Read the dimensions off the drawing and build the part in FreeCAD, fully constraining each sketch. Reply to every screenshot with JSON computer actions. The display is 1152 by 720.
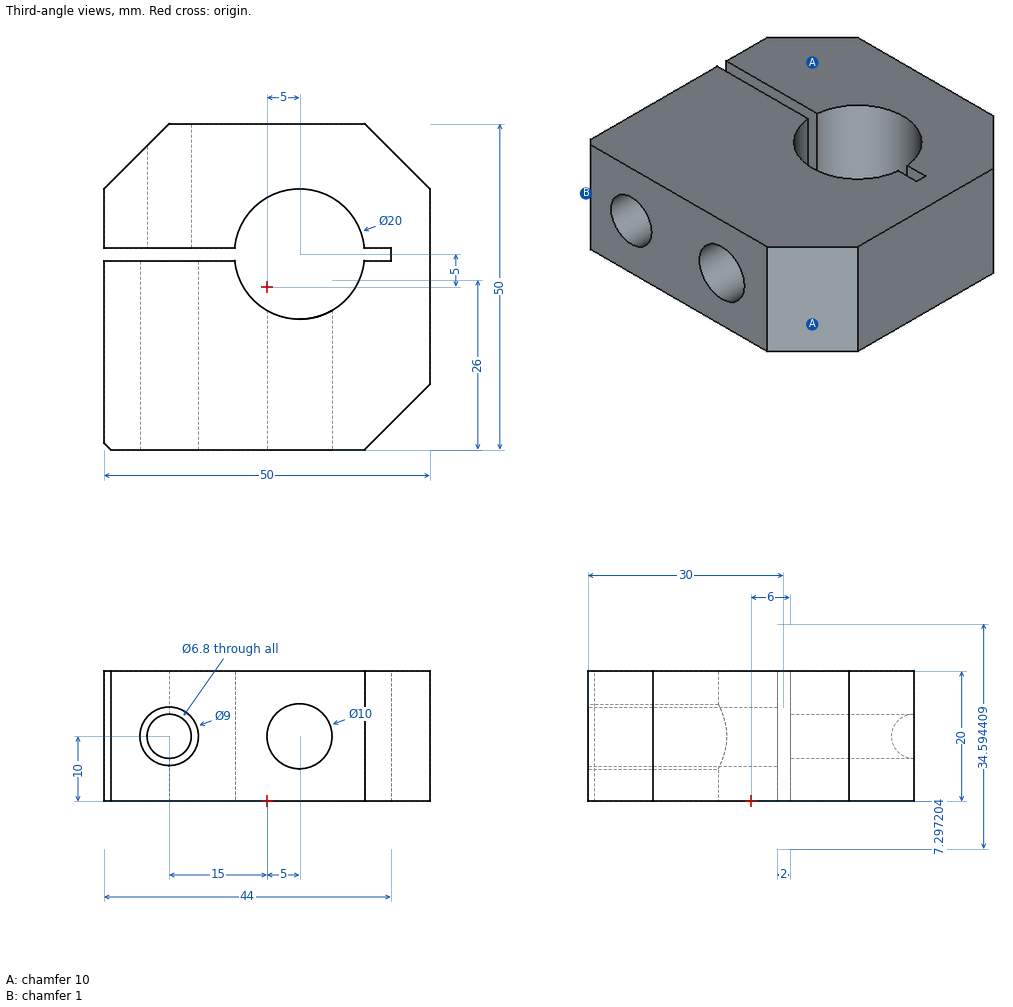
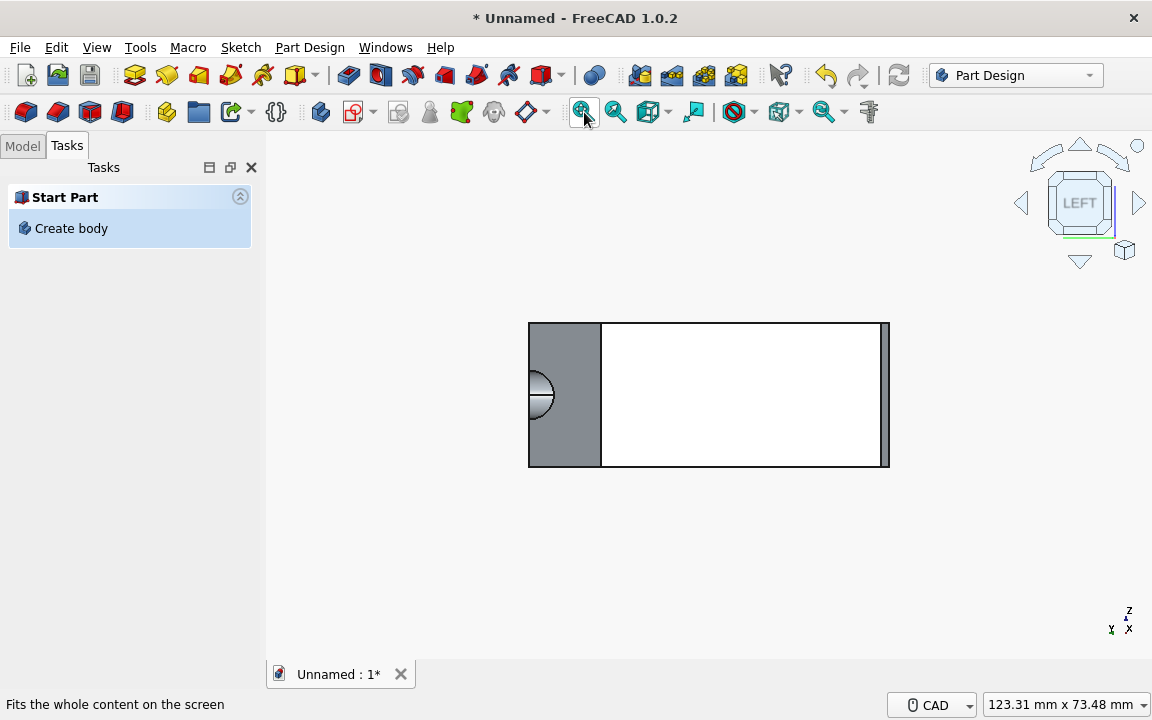
{"action": "left_click", "coordinate": [701, 394]}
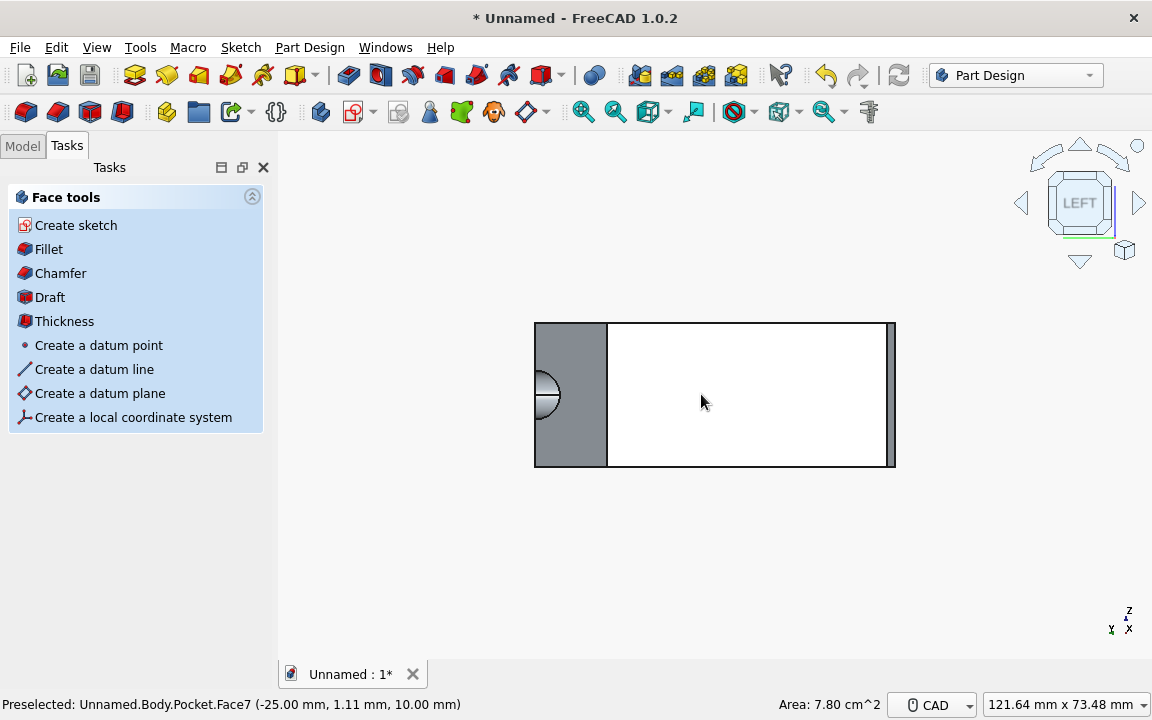
{"action": "left_click", "coordinate": [354, 112]}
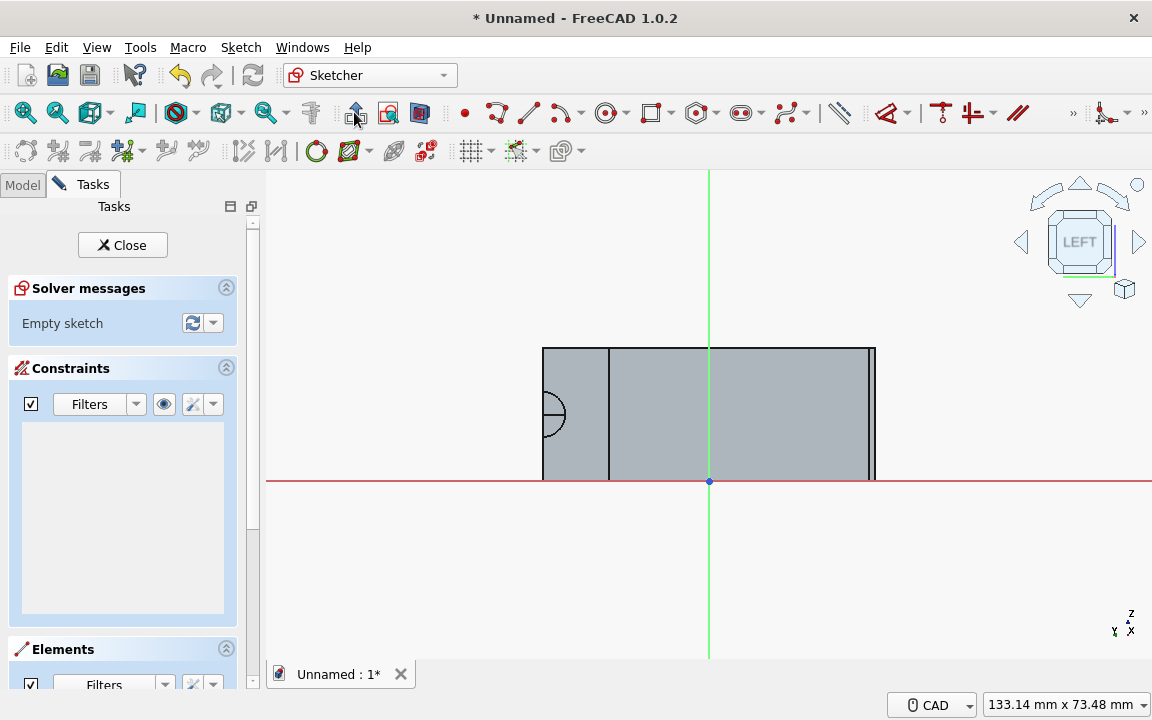
{"action": "left_click", "coordinate": [652, 114]}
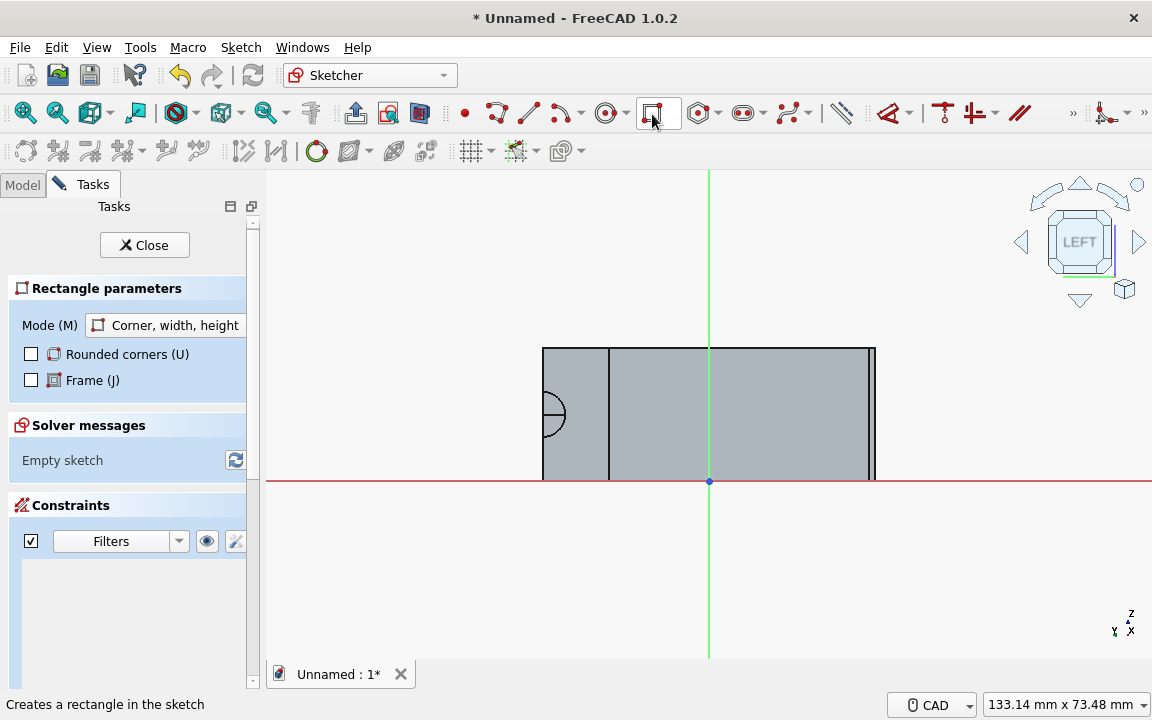
{"action": "left_click", "coordinate": [669, 299]}
{"action": "mouse_move", "coordinate": [682, 530]}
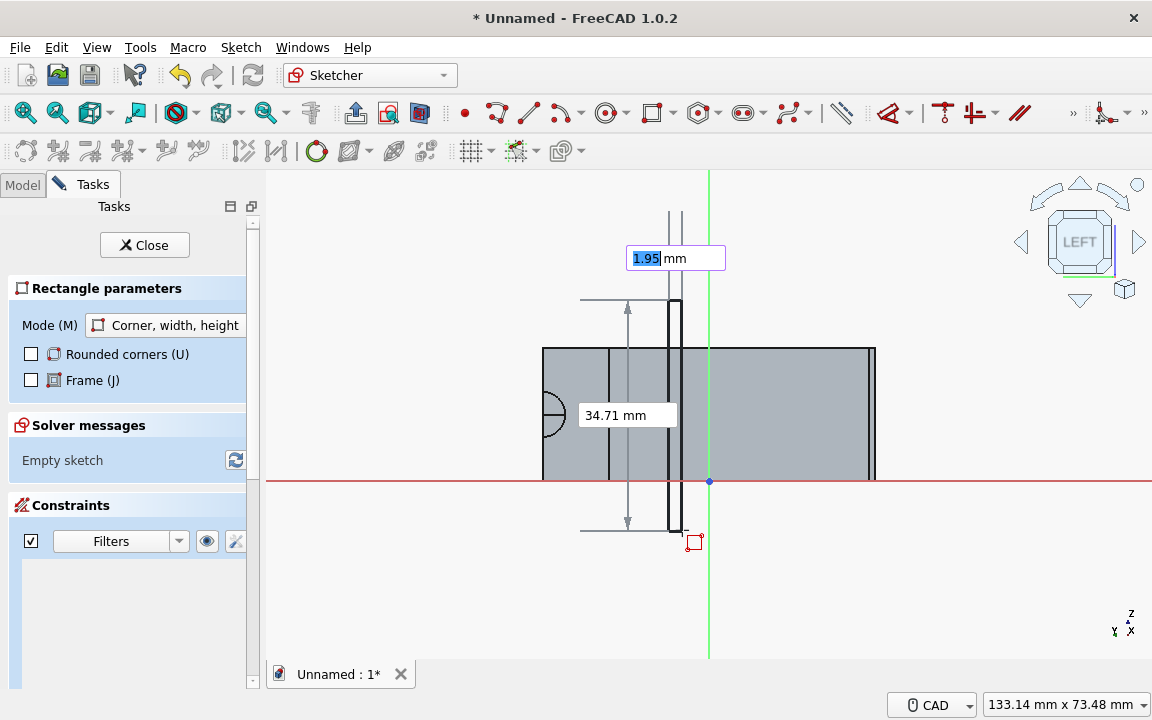
{"action": "type", "text": "2"}
{"action": "key", "text": "Tab"}
{"action": "type", "text": "34.594409"}
{"action": "key", "text": "Return"}
{"action": "key", "text": "Escape"}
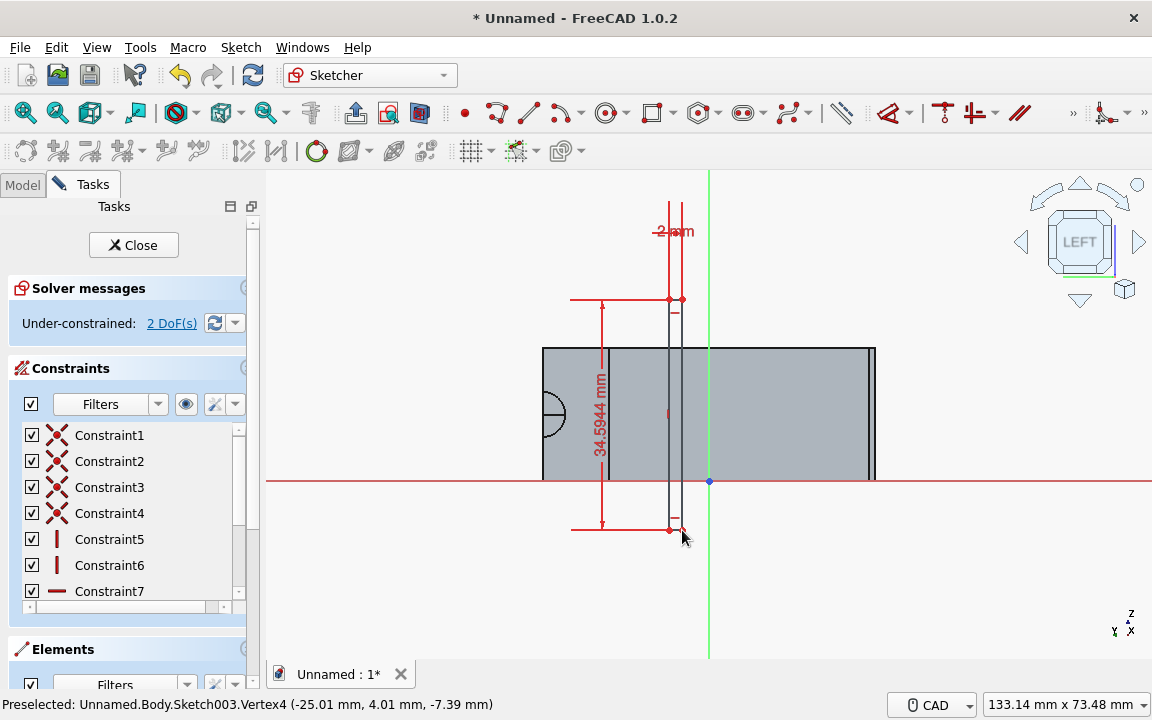
{"action": "left_click", "coordinate": [888, 114]}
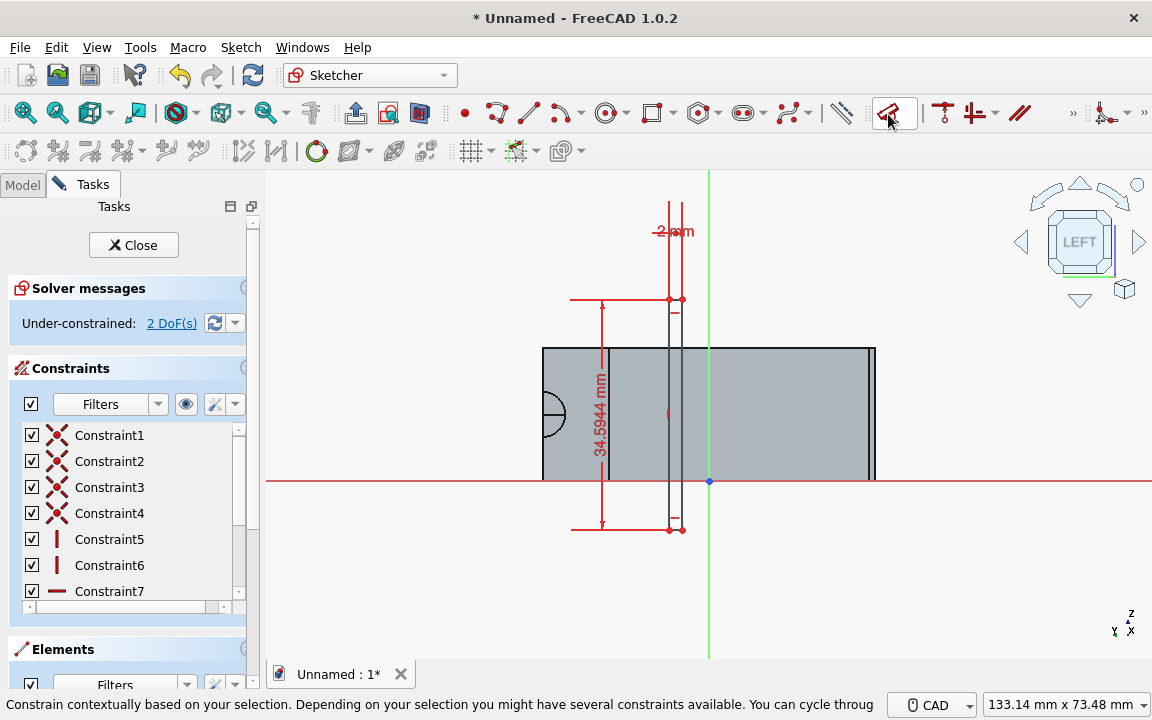
{"action": "left_click", "coordinate": [669, 300]}
{"action": "left_click", "coordinate": [689, 266]}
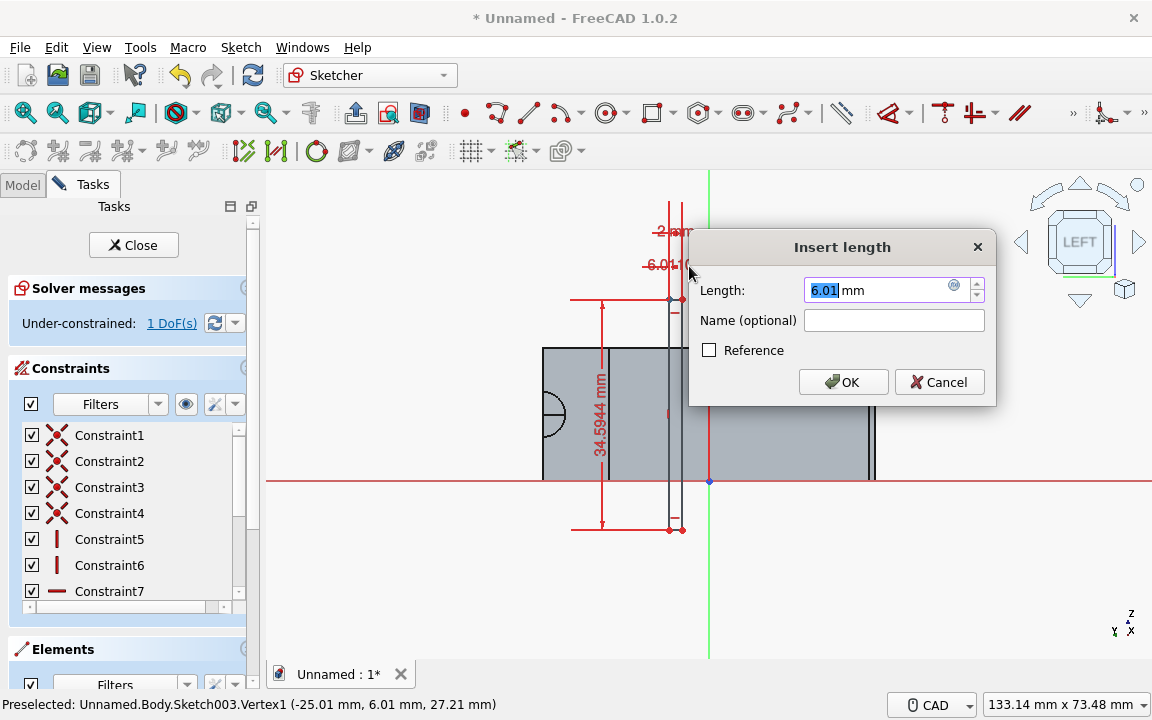
{"action": "type", "text": "6"}
{"action": "key", "text": "Return"}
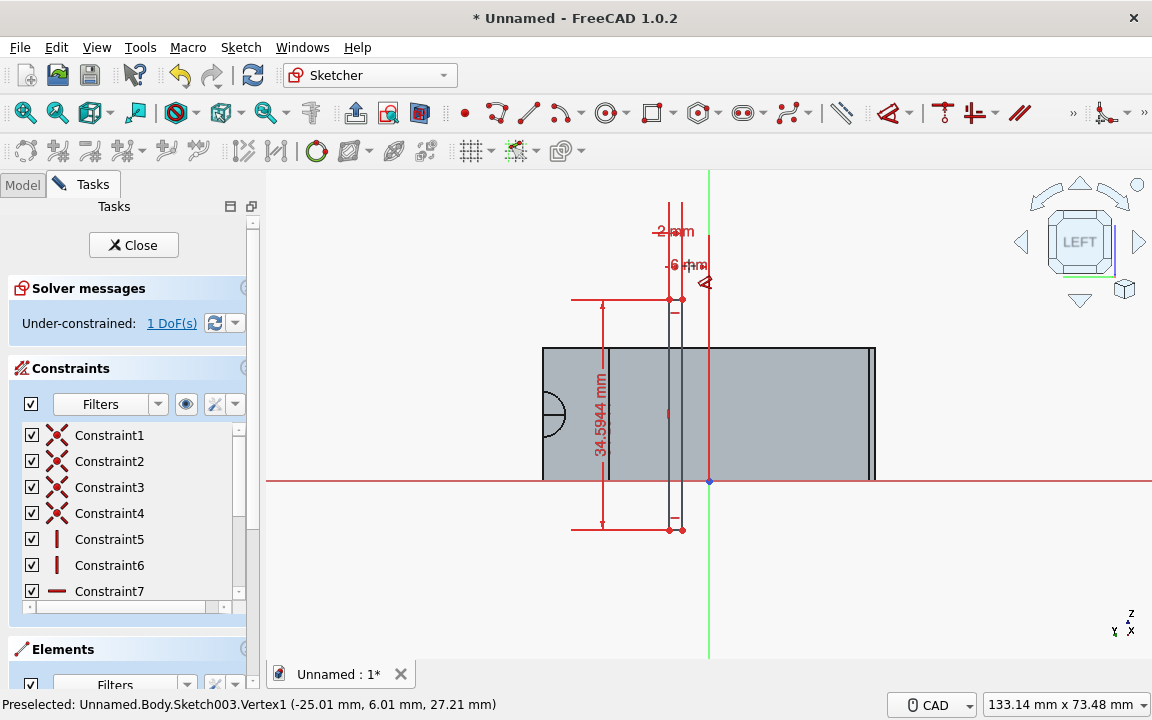
{"action": "left_click", "coordinate": [669, 530]}
{"action": "left_click", "coordinate": [743, 506]}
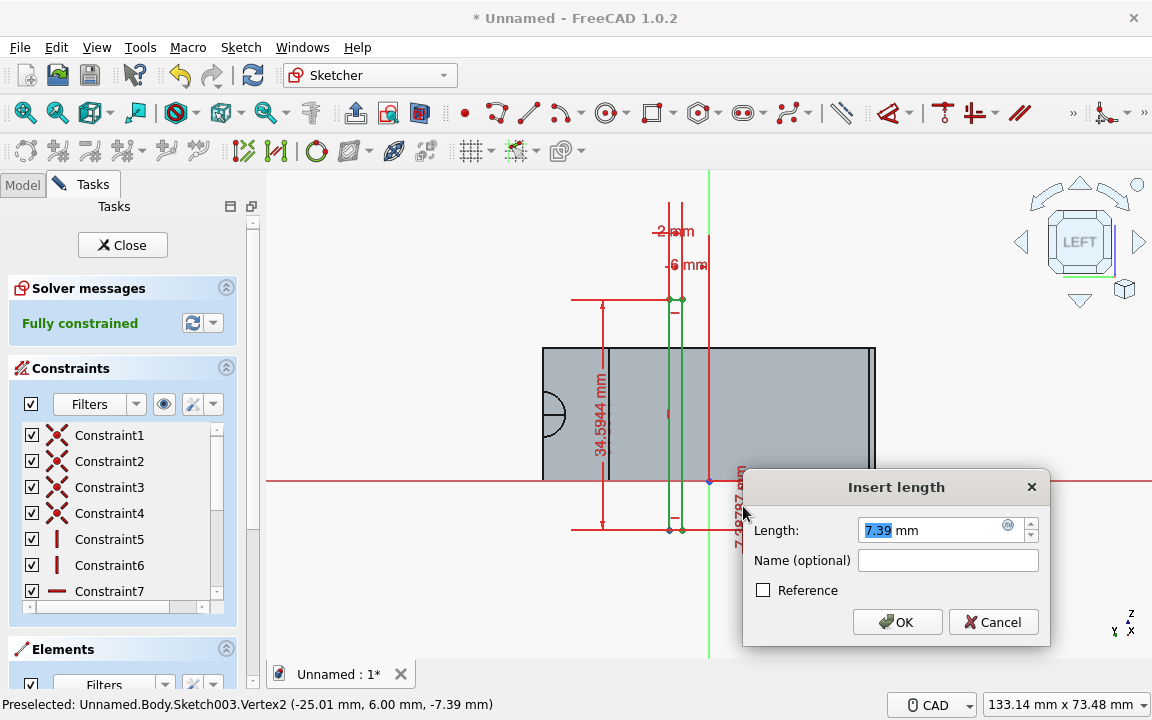
{"action": "type", "text": "7.297204"}
{"action": "key", "text": "Return"}
{"action": "key", "text": "Escape"}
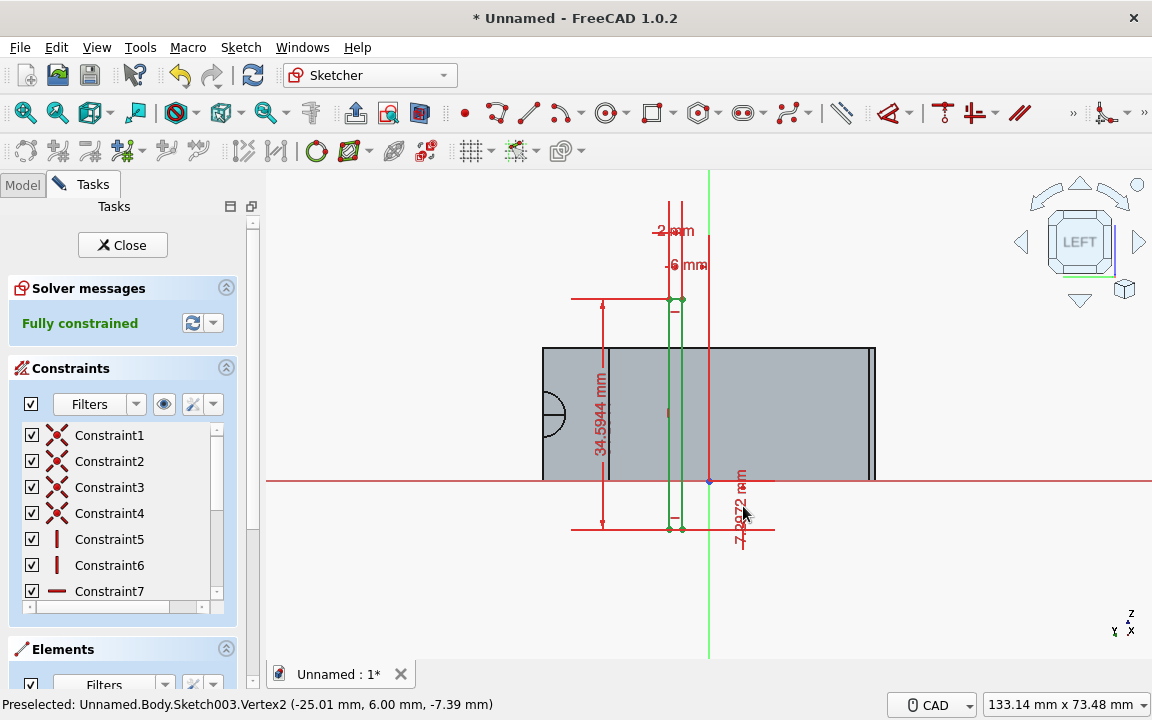
{"action": "left_click", "coordinate": [123, 245]}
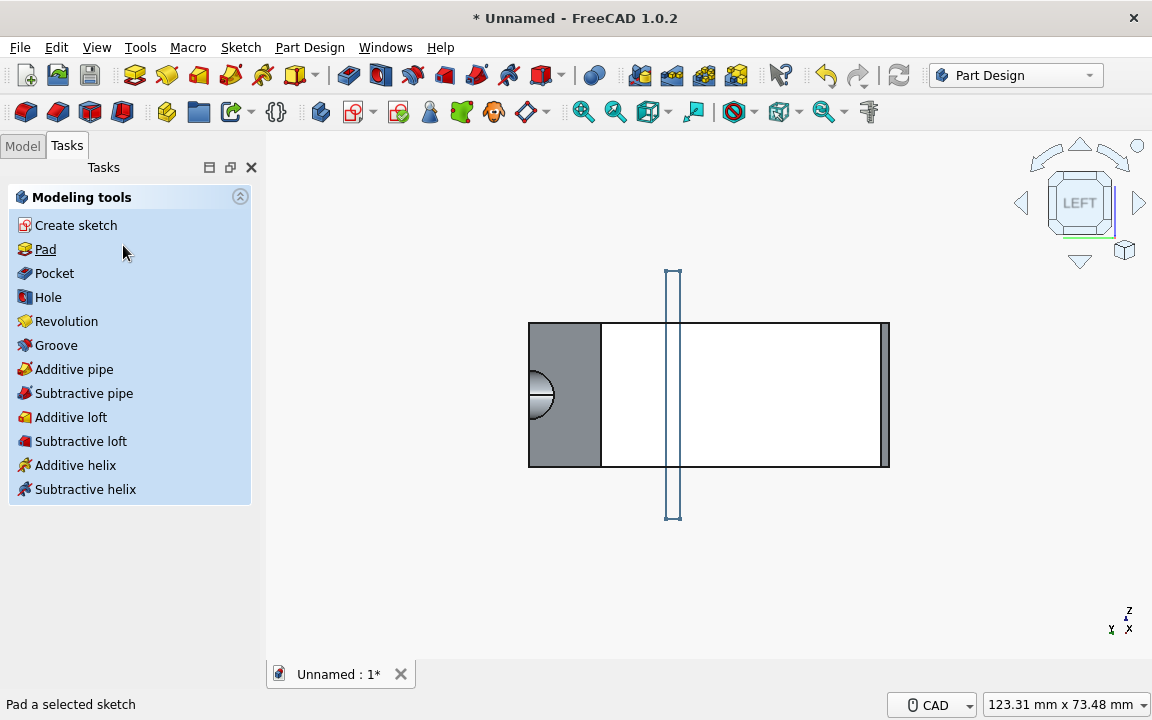
{"action": "left_click", "coordinate": [350, 76]}